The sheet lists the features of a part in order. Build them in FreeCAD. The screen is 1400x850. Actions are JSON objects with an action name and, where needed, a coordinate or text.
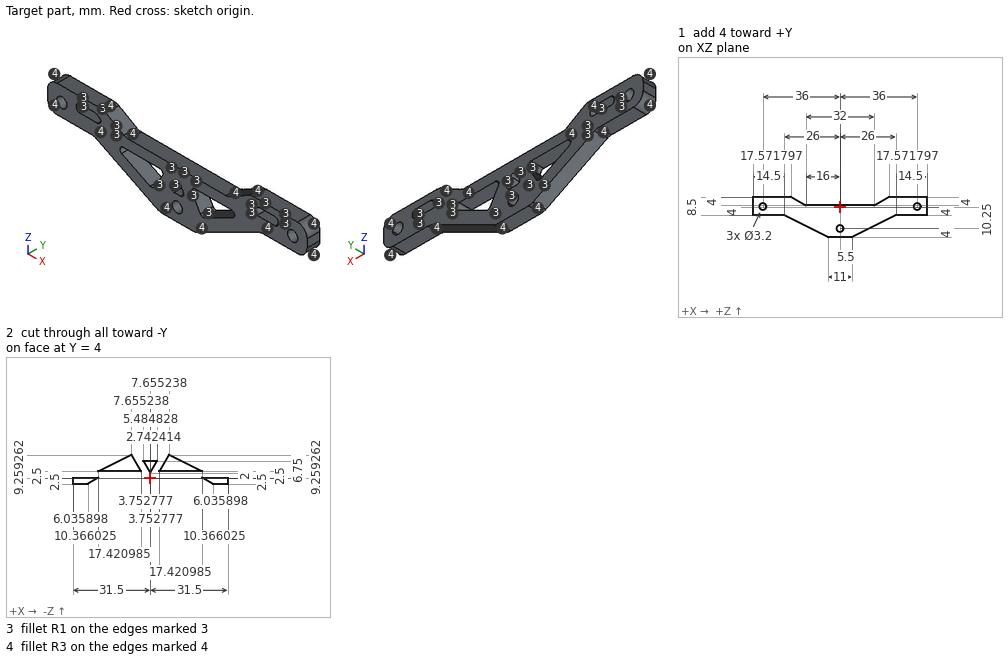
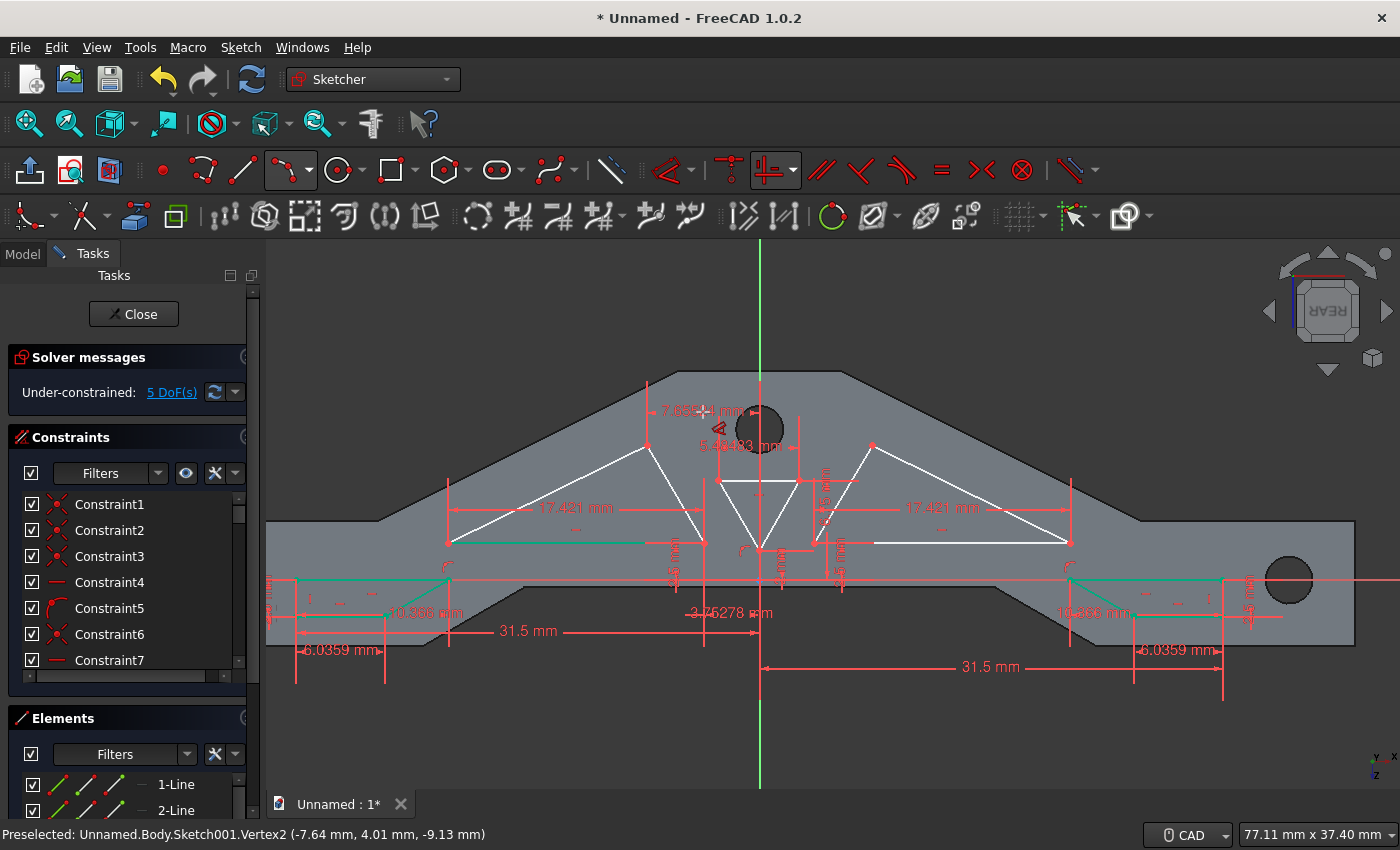
{"action": "left_click", "coordinate": [647, 446]}
{"action": "left_click", "coordinate": [613, 482]}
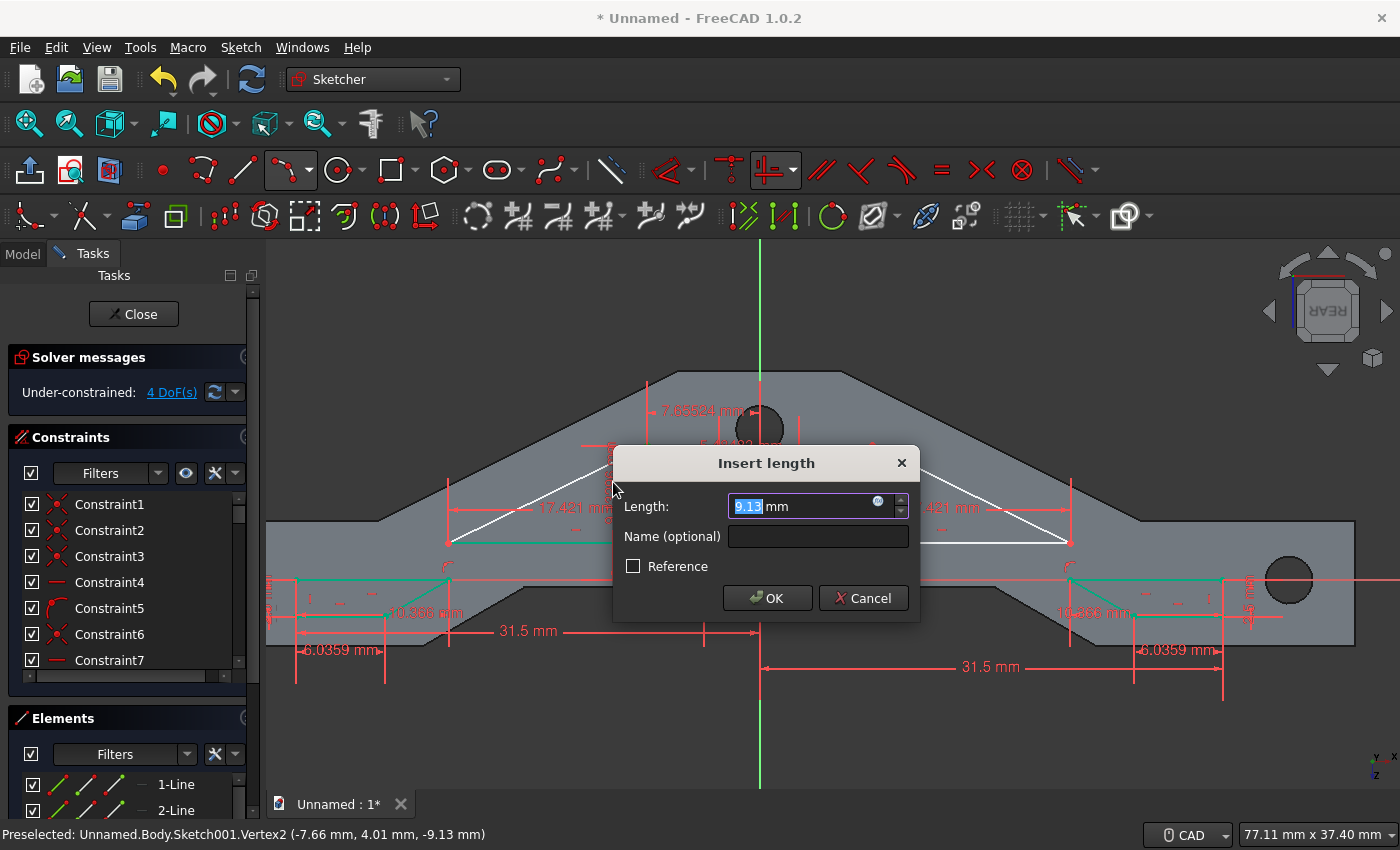
{"action": "type", "text": "9.259262"}
{"action": "key", "text": "Return"}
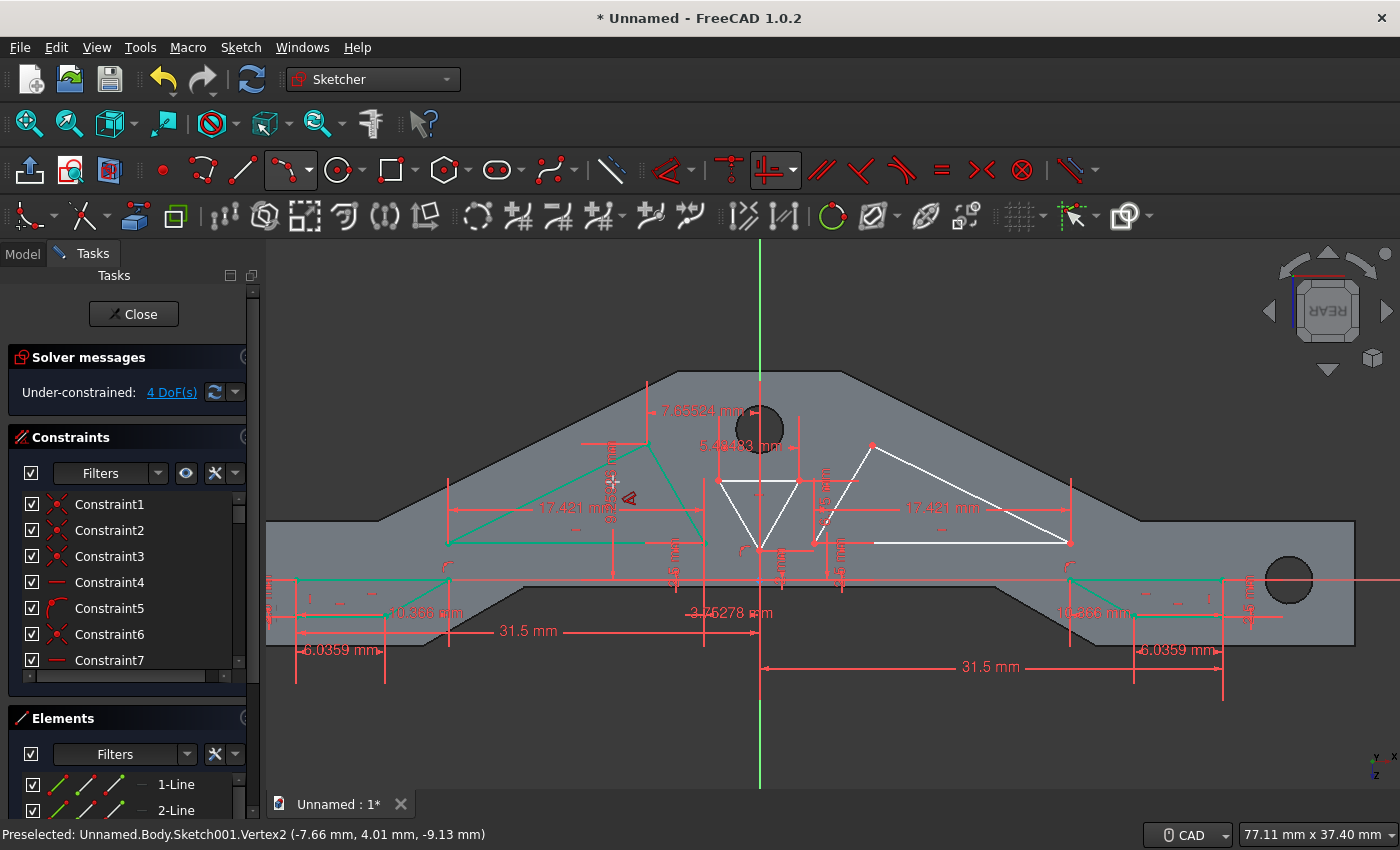
{"action": "left_click", "coordinate": [799, 481]}
{"action": "left_click", "coordinate": [780, 638]}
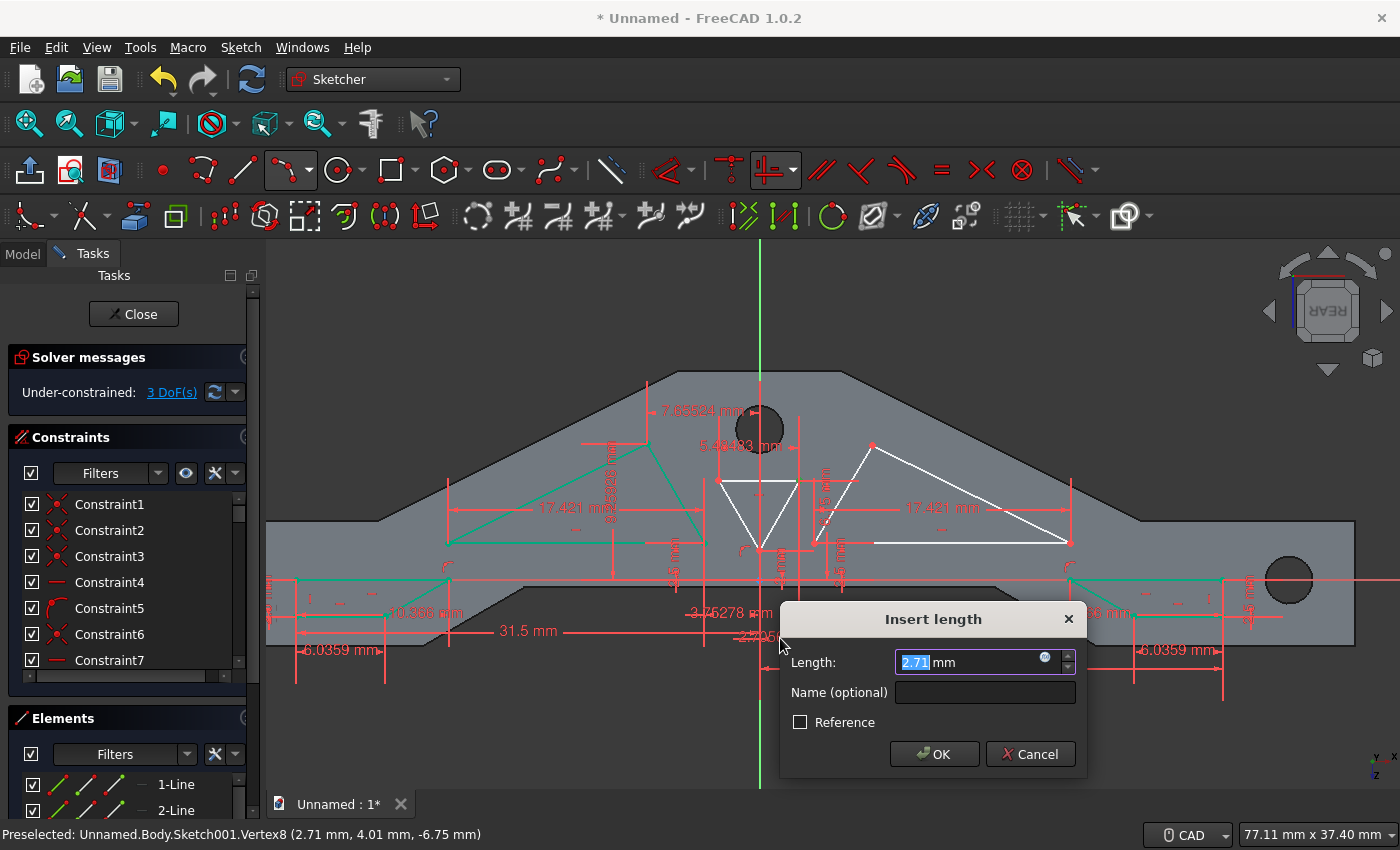
{"action": "type", "text": "2.742414"}
{"action": "key", "text": "Return"}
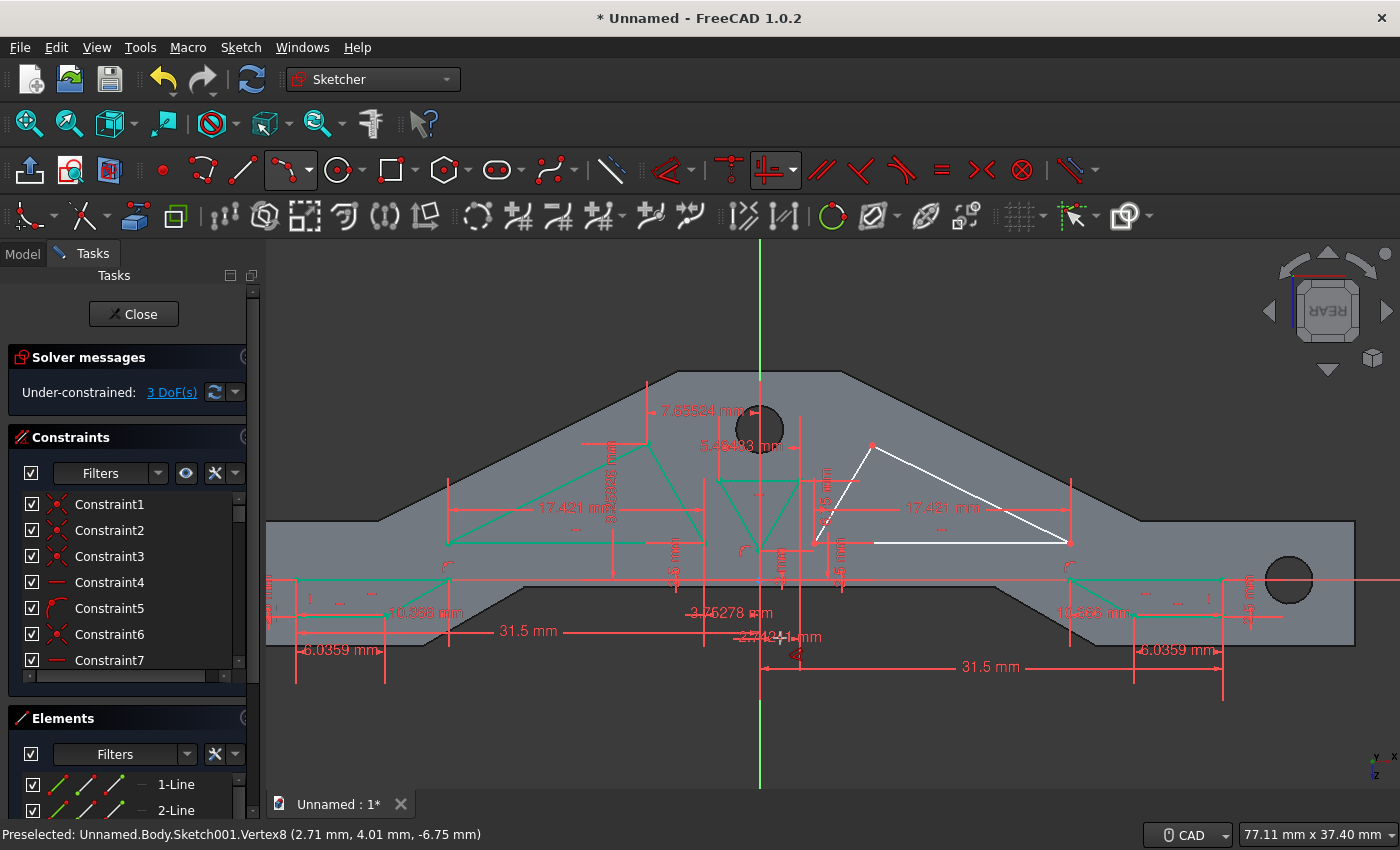
{"action": "left_click", "coordinate": [814, 543]}
{"action": "left_click", "coordinate": [806, 614]}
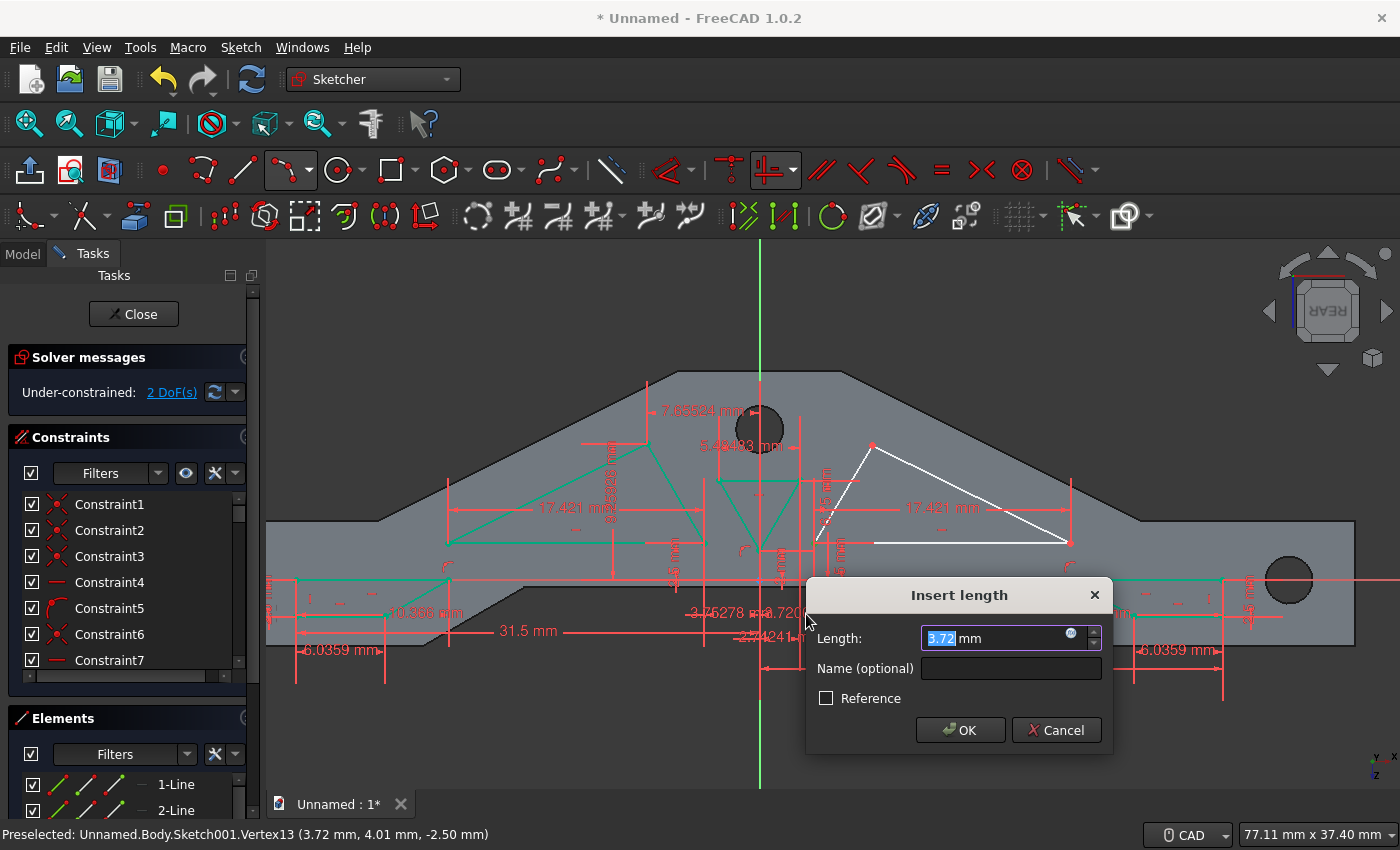
{"action": "type", "text": "3.752777"}
{"action": "key", "text": "Return"}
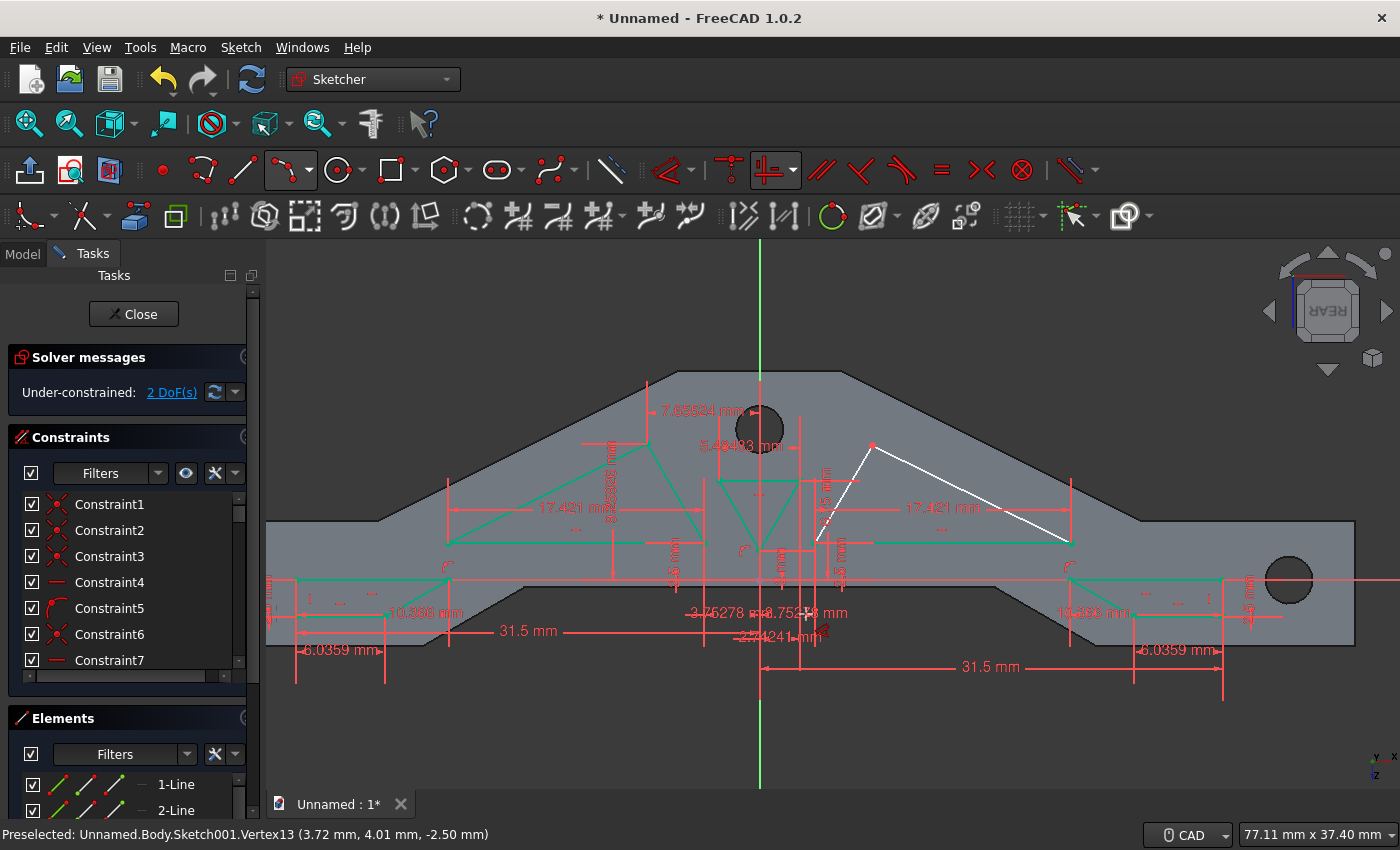
{"action": "left_click", "coordinate": [873, 446]}
{"action": "left_click", "coordinate": [816, 412]}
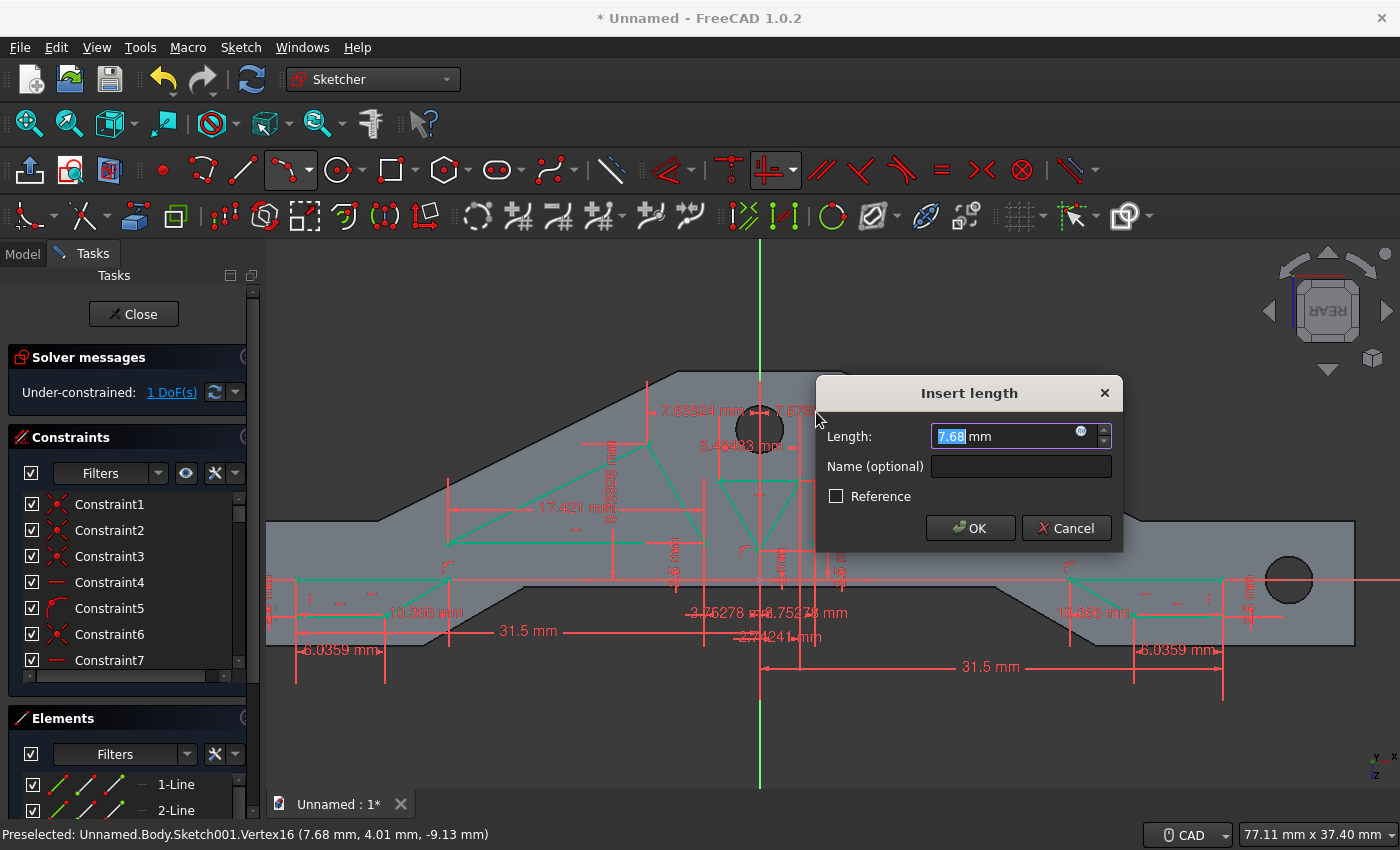
{"action": "type", "text": "7.655238"}
{"action": "key", "text": "Return"}